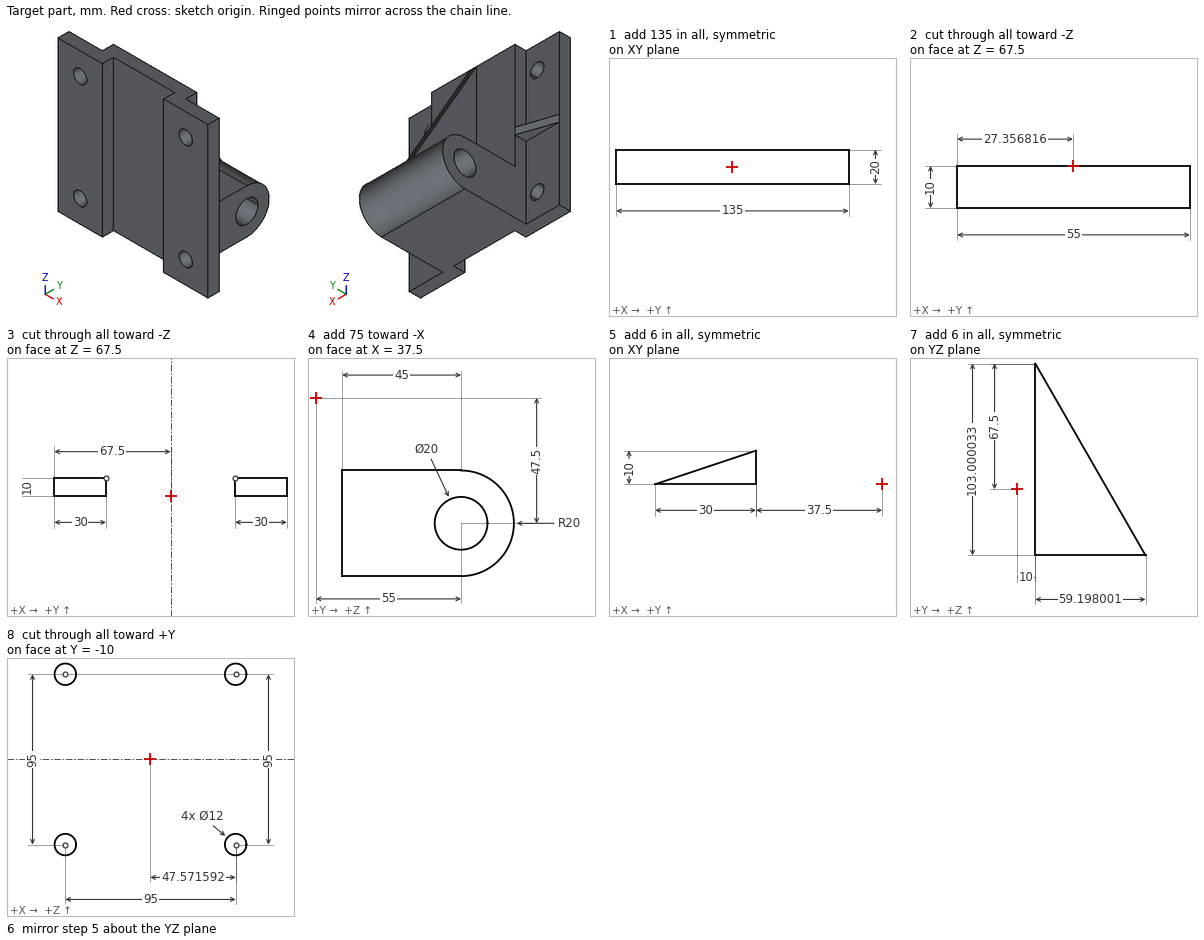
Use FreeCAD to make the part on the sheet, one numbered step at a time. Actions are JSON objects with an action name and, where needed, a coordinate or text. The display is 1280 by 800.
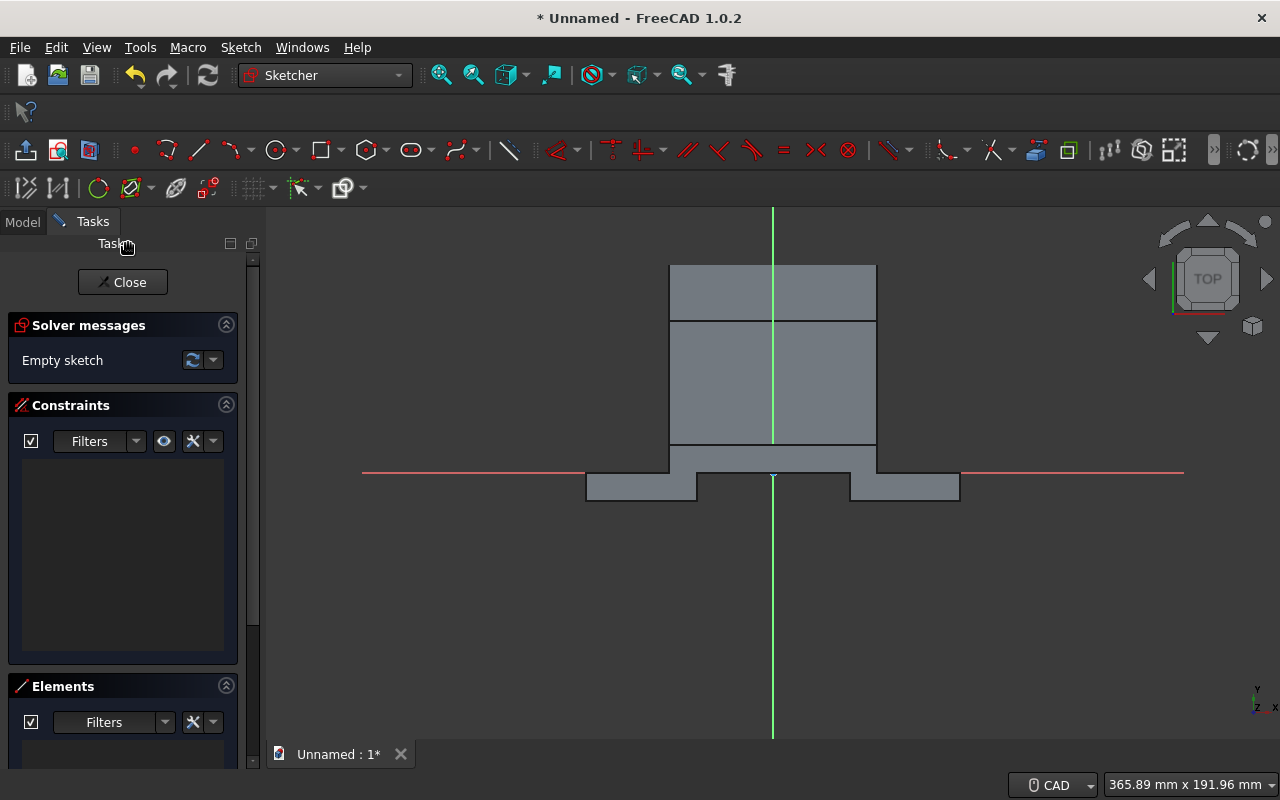
{"action": "left_click", "coordinate": [90, 150]}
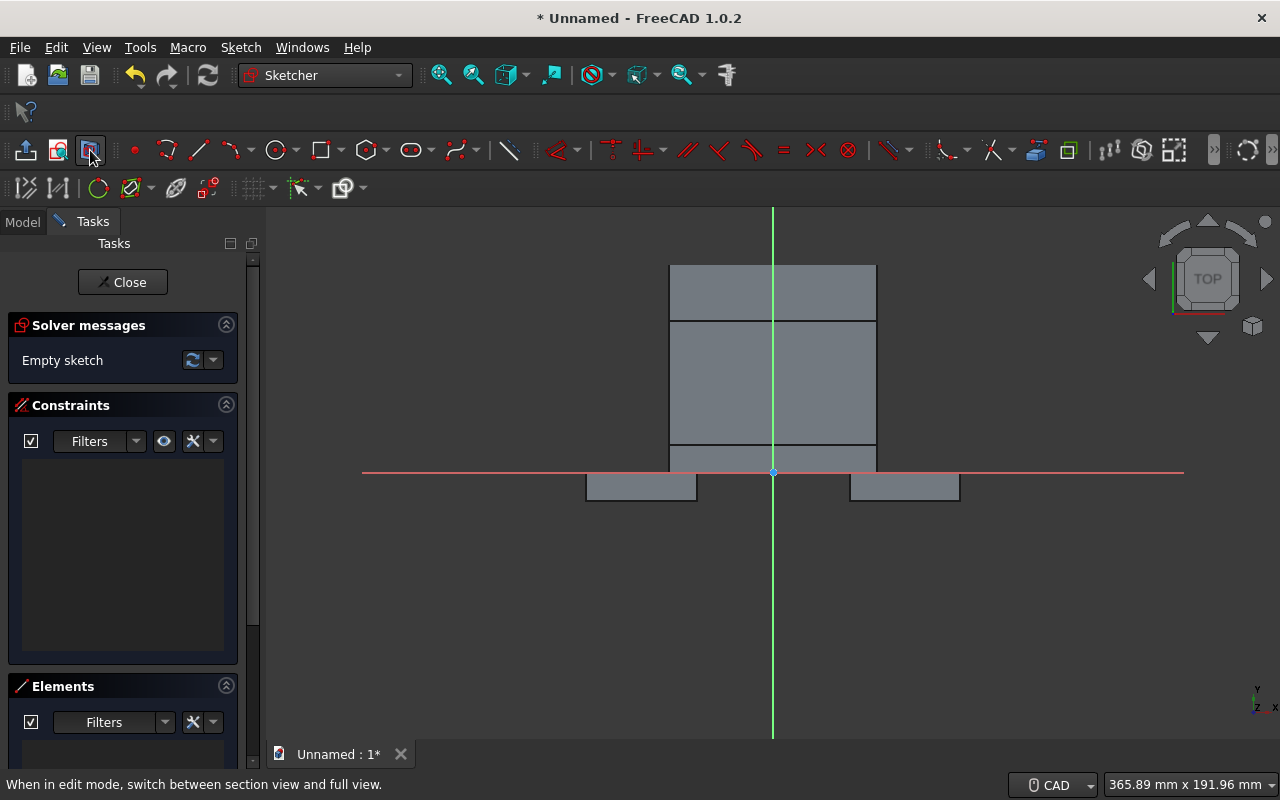
{"action": "scroll", "coordinate": [669, 453], "scroll_direction": "up", "scroll_amount": 6}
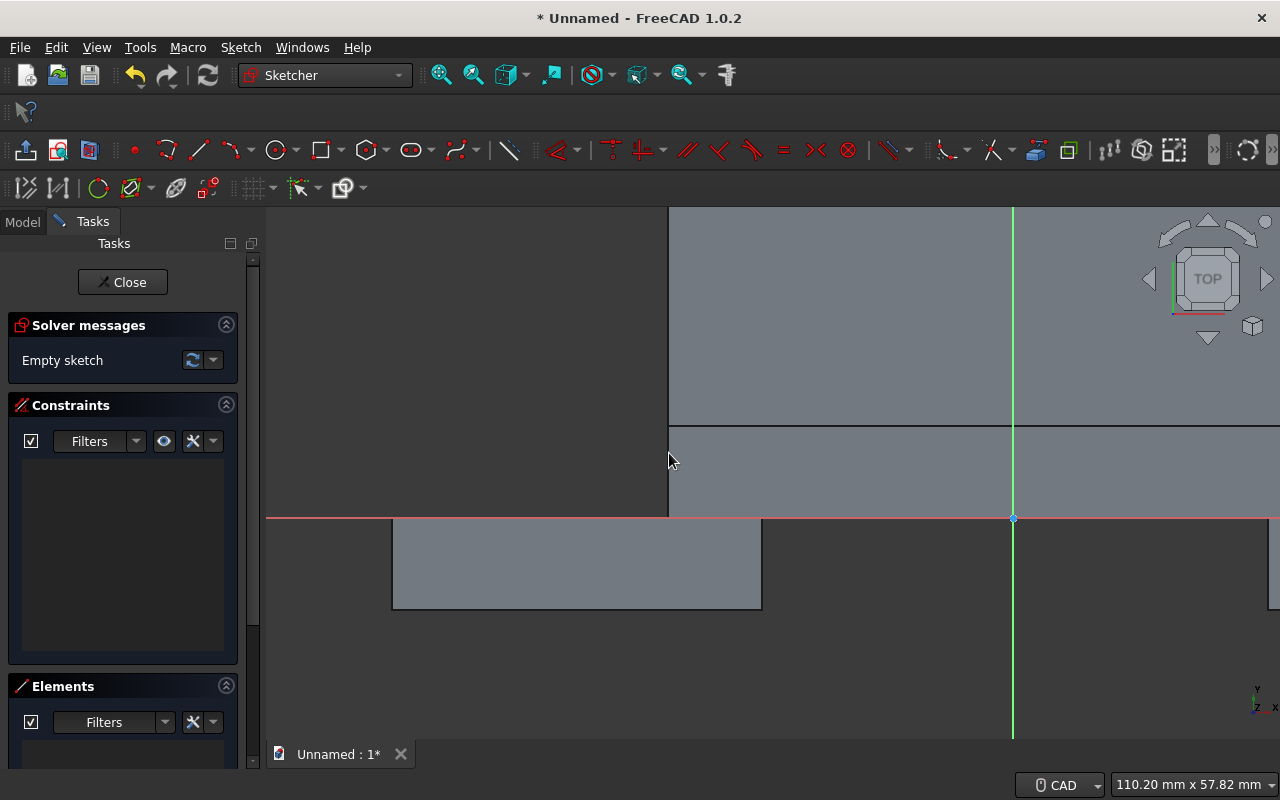
{"action": "key", "text": "g m"}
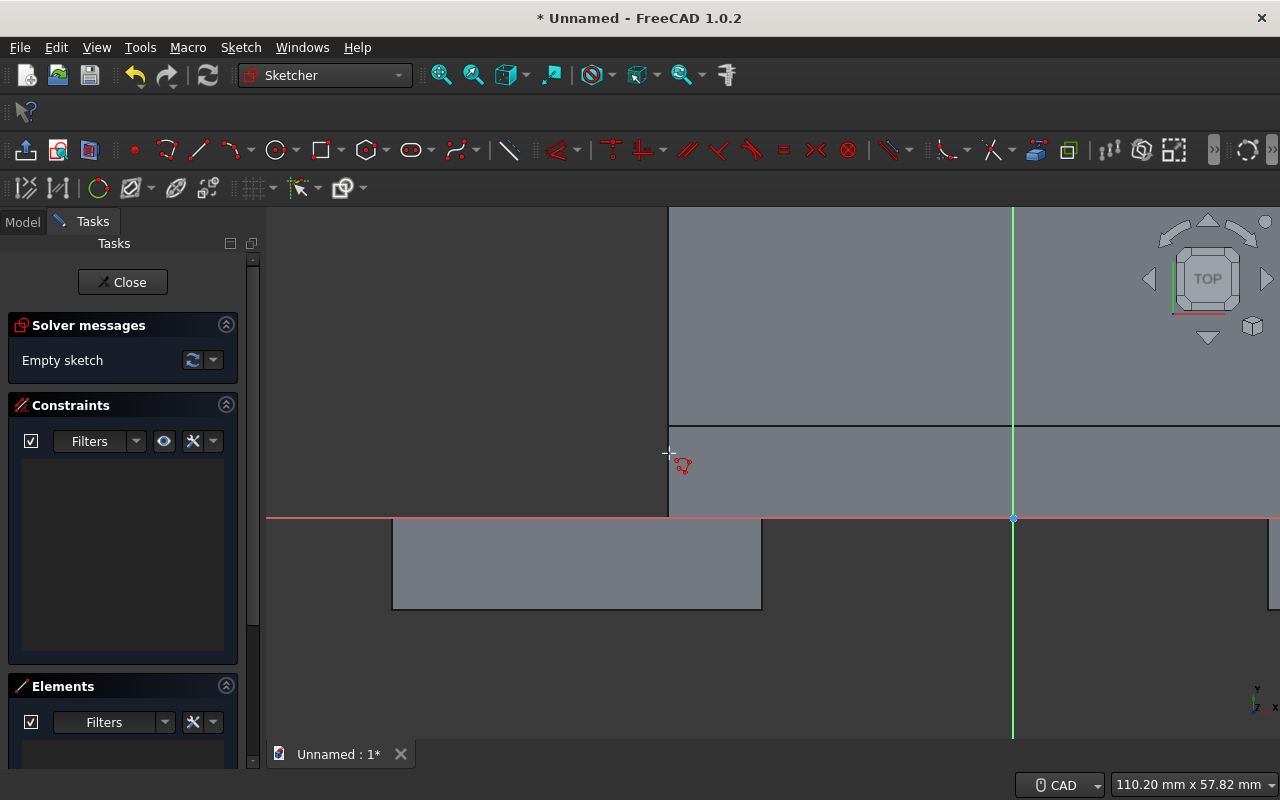
{"action": "left_click", "coordinate": [668, 518]}
{"action": "left_click", "coordinate": [668, 426]}
{"action": "left_click", "coordinate": [392, 509]}
{"action": "left_click", "coordinate": [668, 518]}
{"action": "key", "text": "Escape"}
{"action": "key", "text": "Escape"}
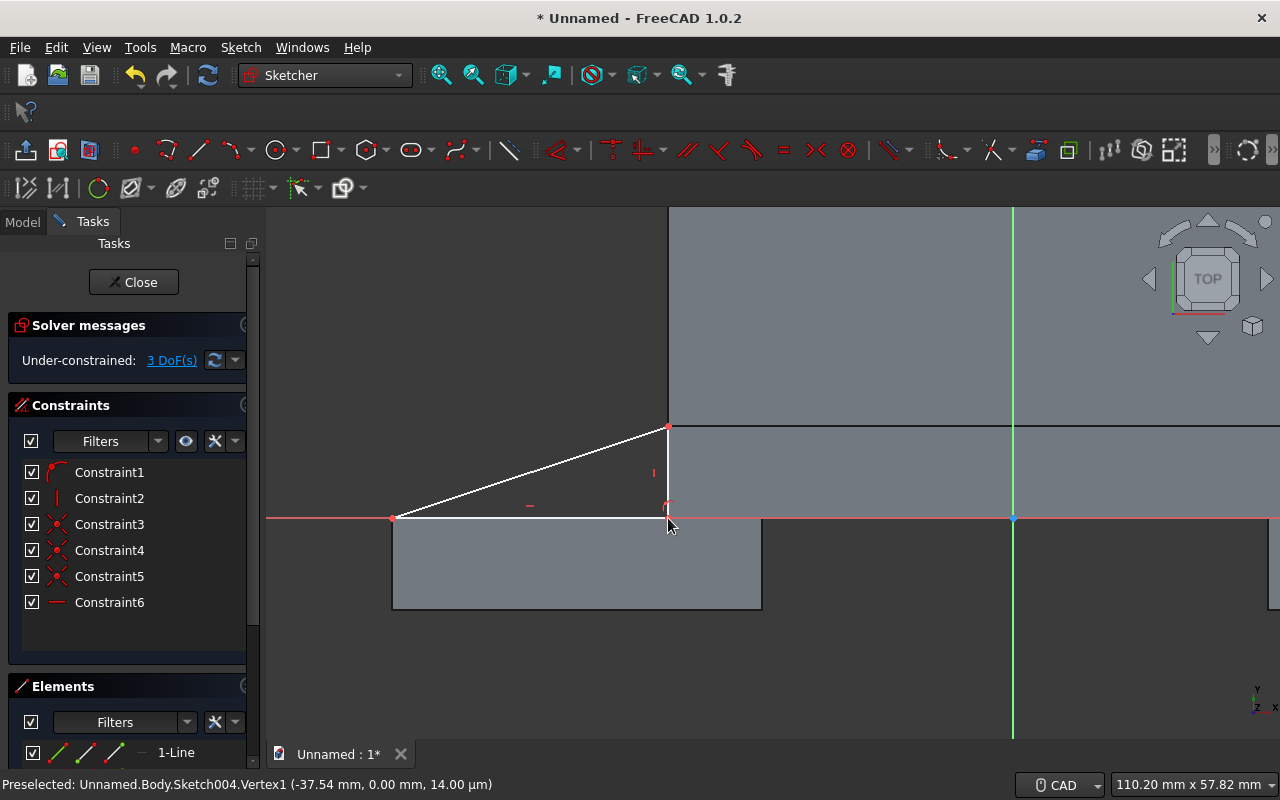
{"action": "left_click", "coordinate": [556, 150]}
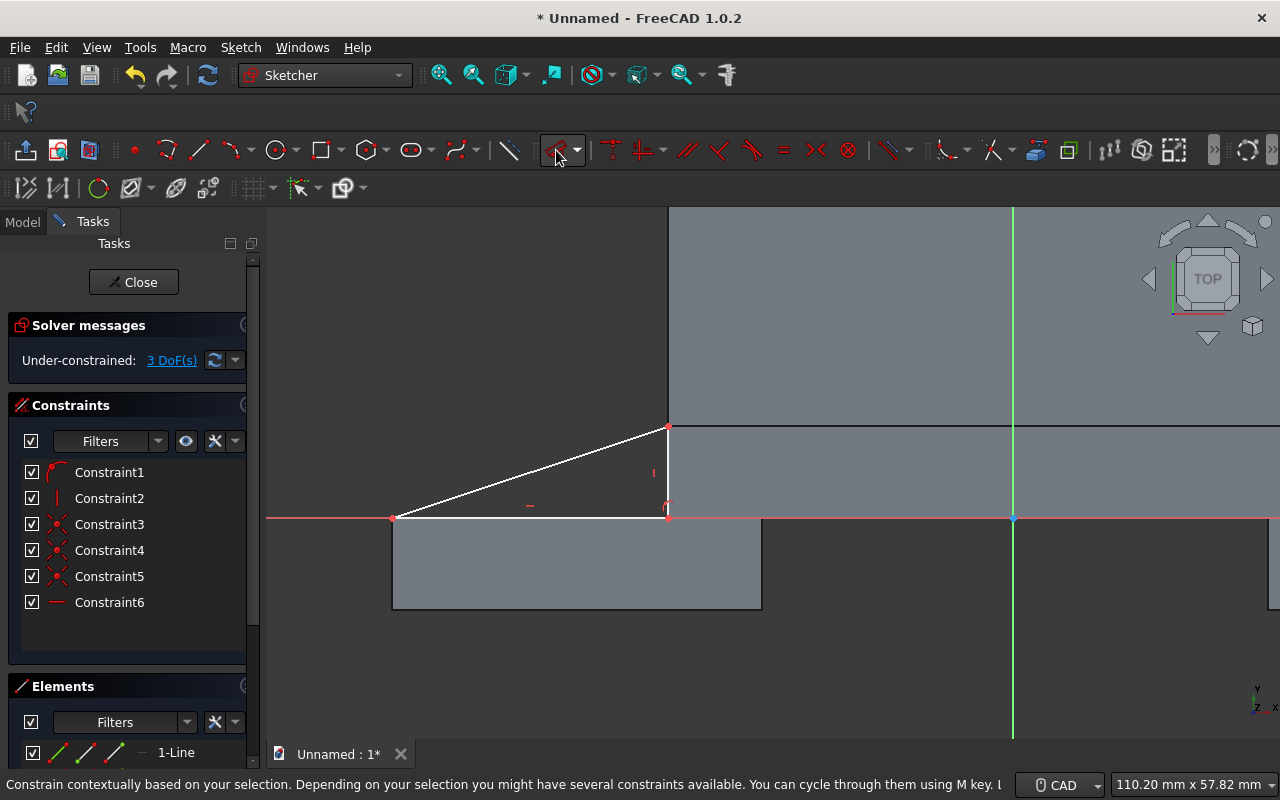
{"action": "left_click", "coordinate": [668, 491]}
{"action": "left_click", "coordinate": [634, 473]}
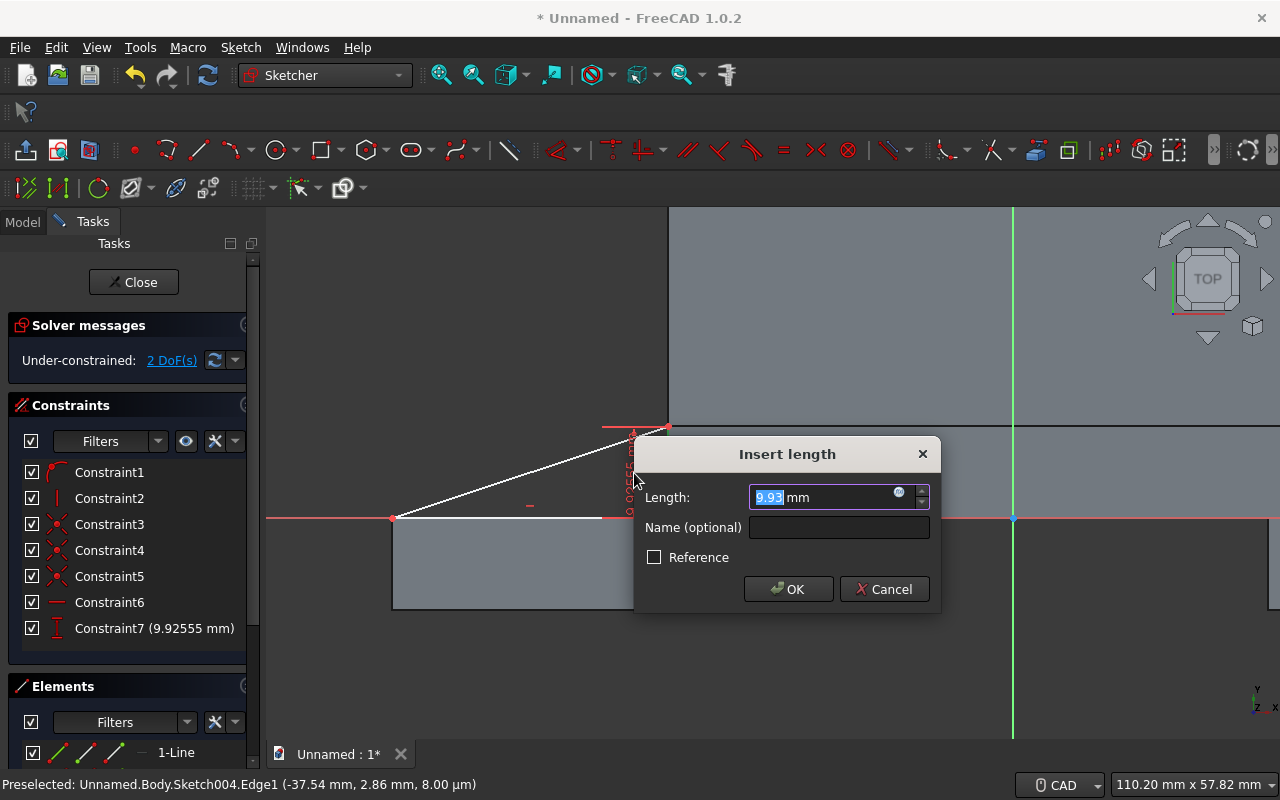
{"action": "type", "text": "10"}
{"action": "key", "text": "Return"}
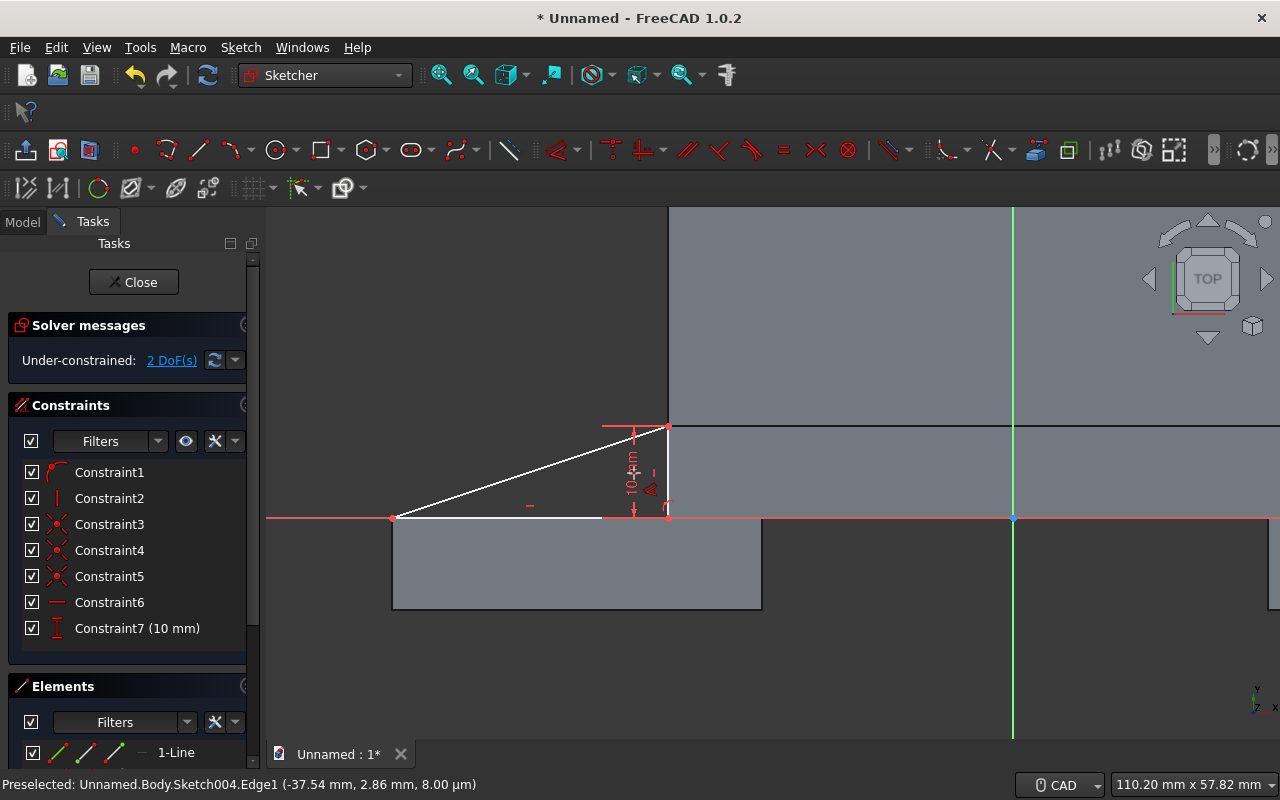
{"action": "left_click", "coordinate": [475, 518]}
{"action": "left_click", "coordinate": [530, 552]}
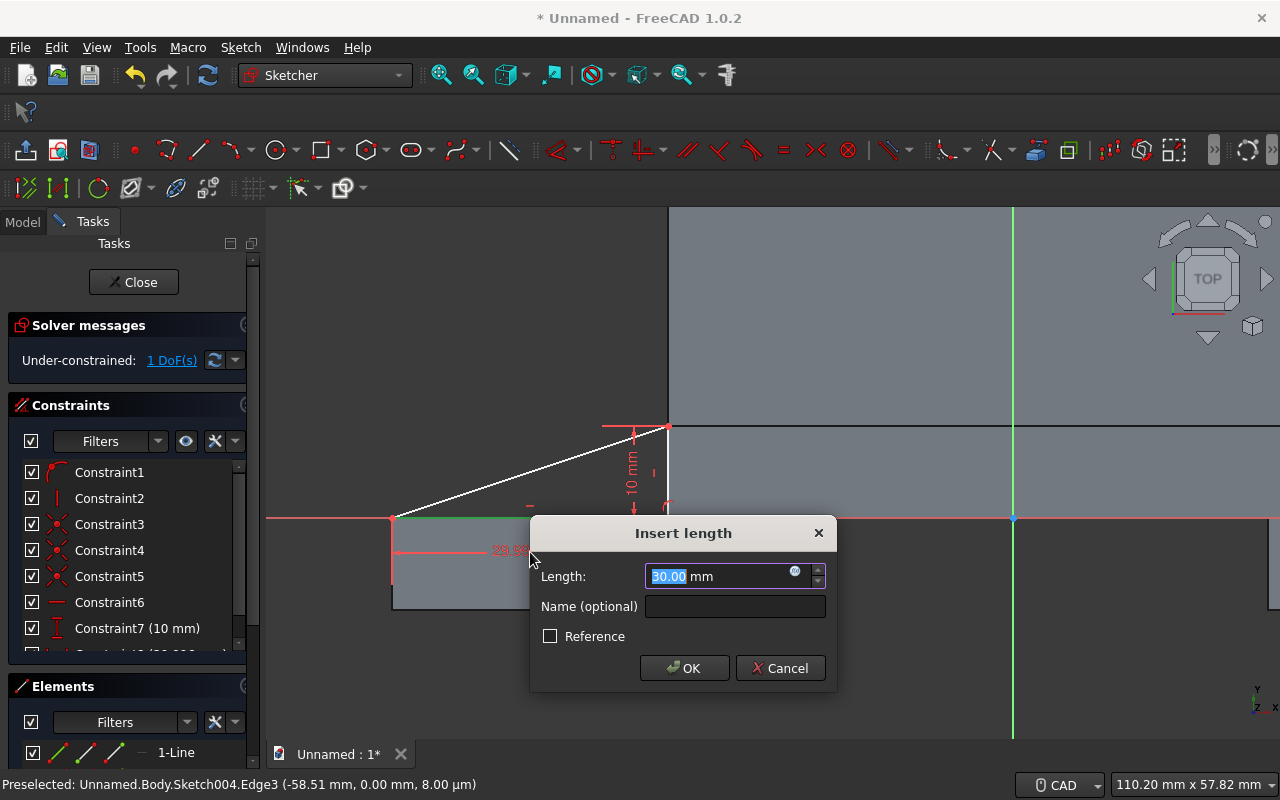
{"action": "type", "text": "30"}
{"action": "key", "text": "Return"}